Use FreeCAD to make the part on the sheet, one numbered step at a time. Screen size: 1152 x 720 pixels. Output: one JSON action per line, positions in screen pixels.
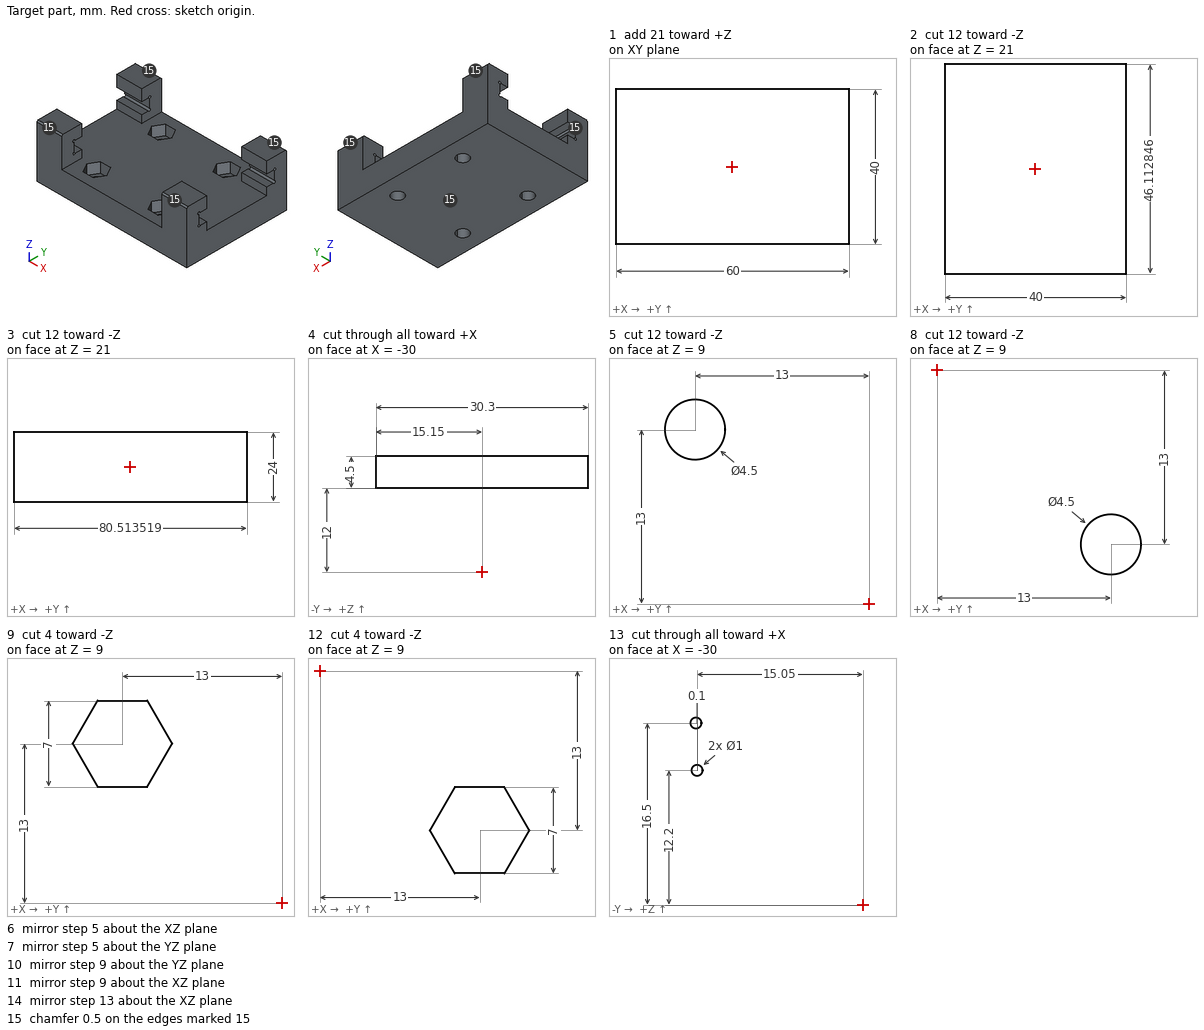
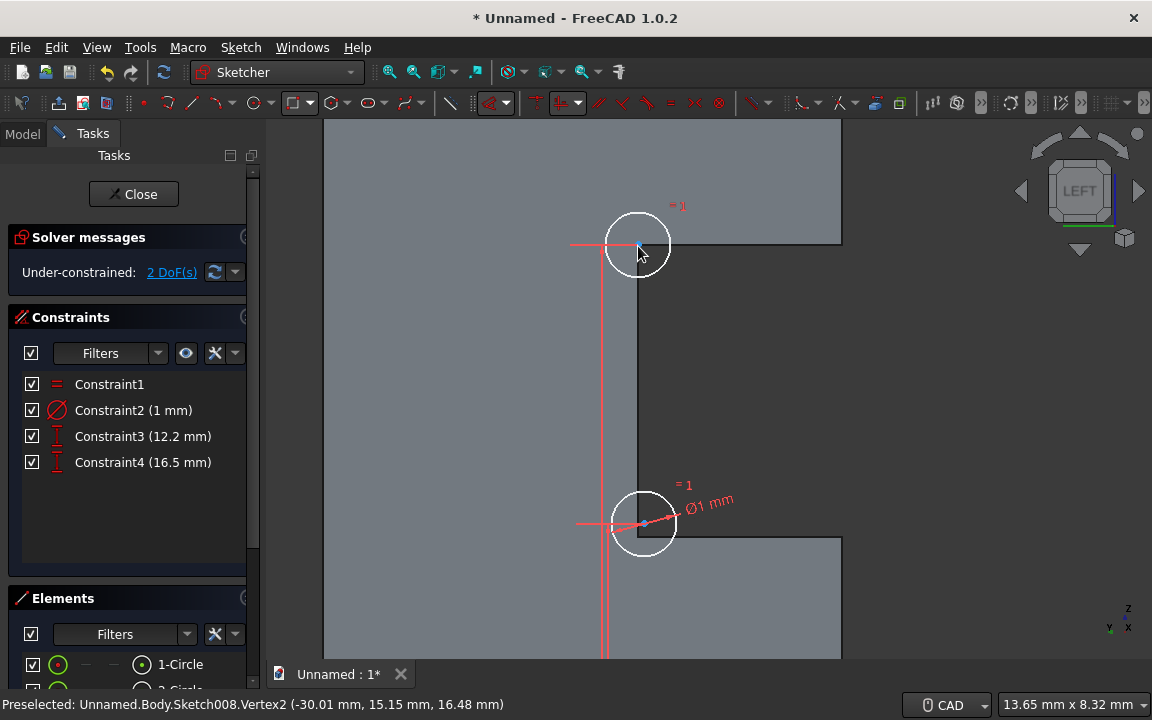
{"action": "scroll", "coordinate": [644, 524], "scroll_direction": "up", "scroll_amount": 10}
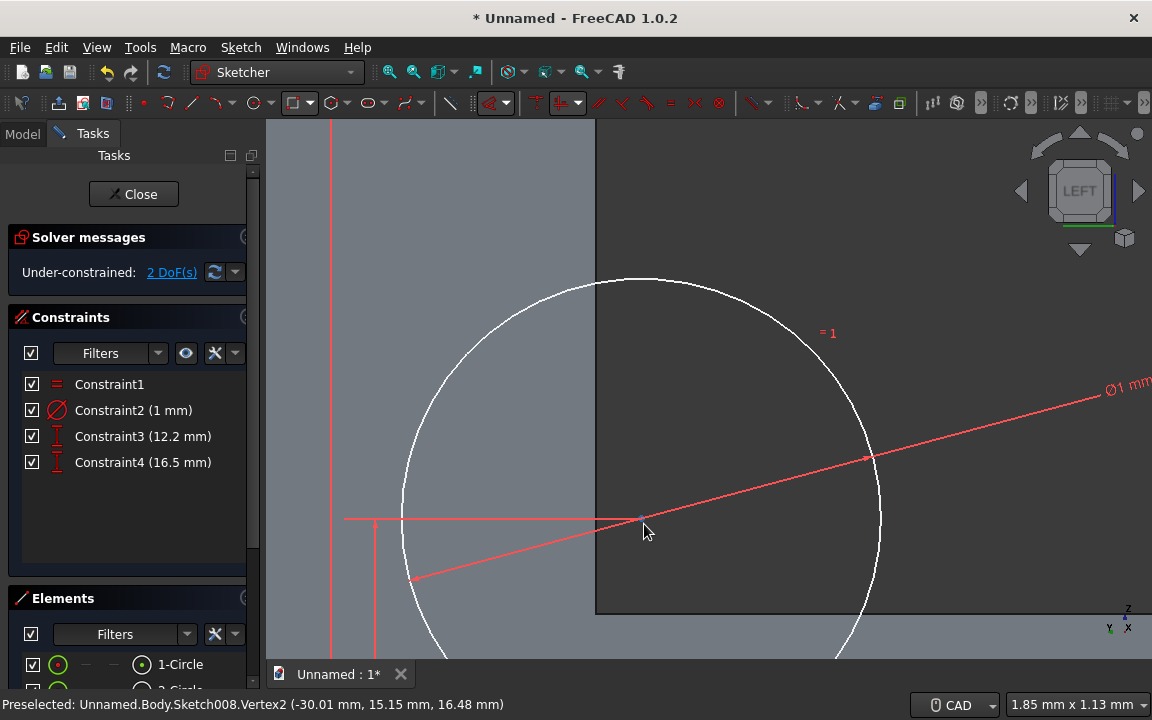
{"action": "left_click", "coordinate": [641, 519]}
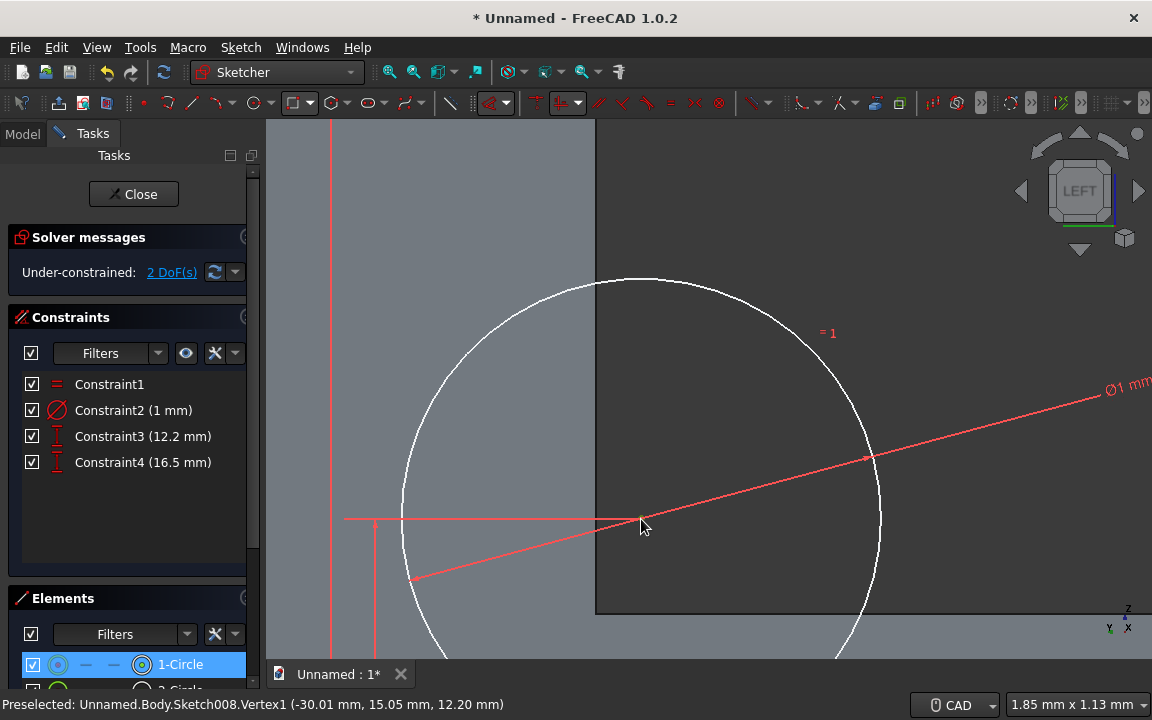
{"action": "scroll", "coordinate": [644, 530], "scroll_direction": "down", "scroll_amount": 10}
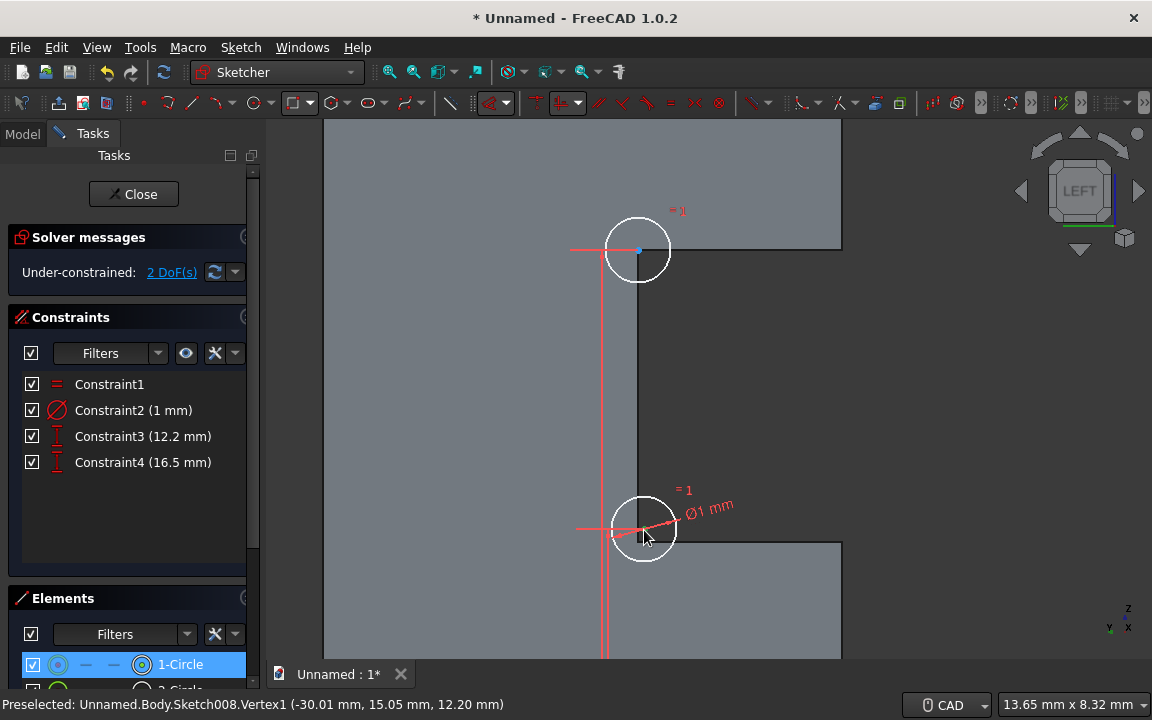
{"action": "scroll", "coordinate": [638, 250], "scroll_direction": "up", "scroll_amount": 10}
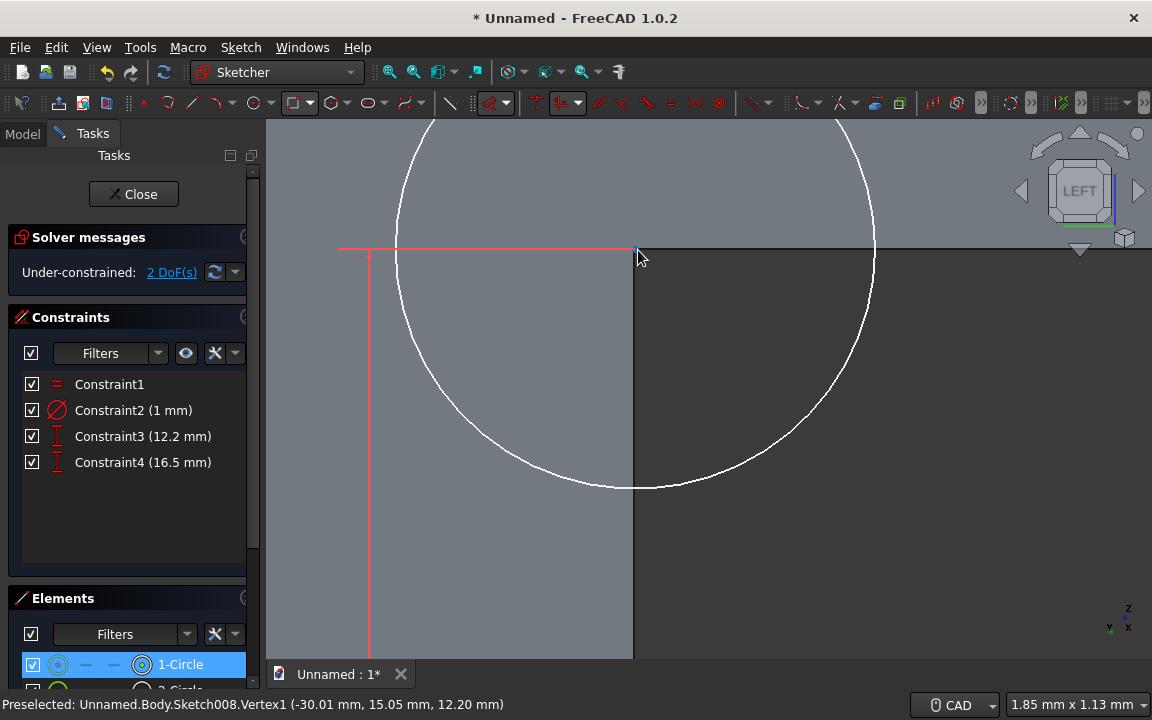
{"action": "left_click", "coordinate": [635, 249]}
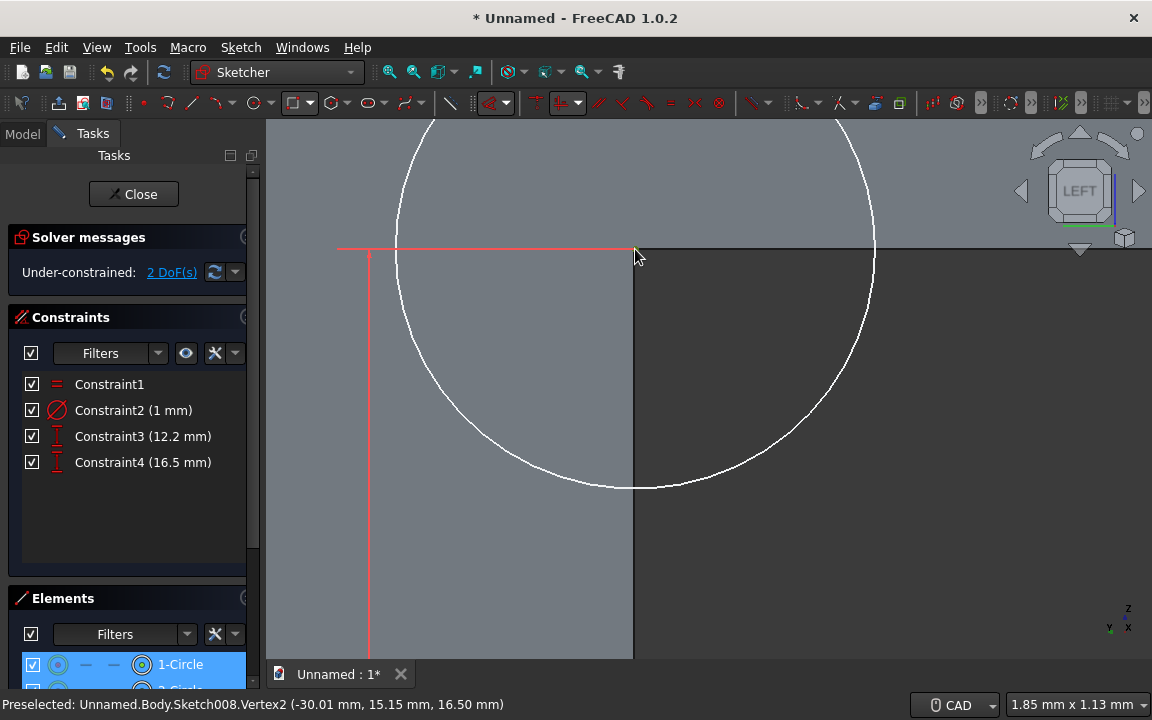
{"action": "key", "text": "l"}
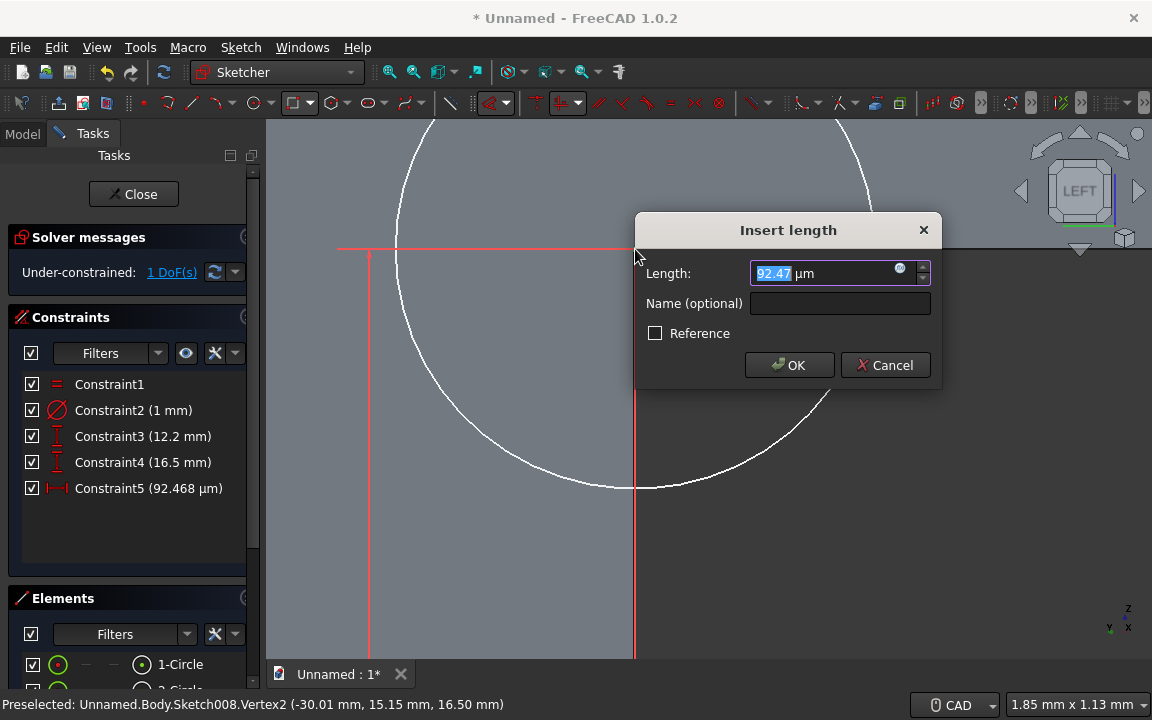
{"action": "key", "text": "ctrl+a"}
{"action": "type", "text": "0.1 mm"}
{"action": "key", "text": "Return"}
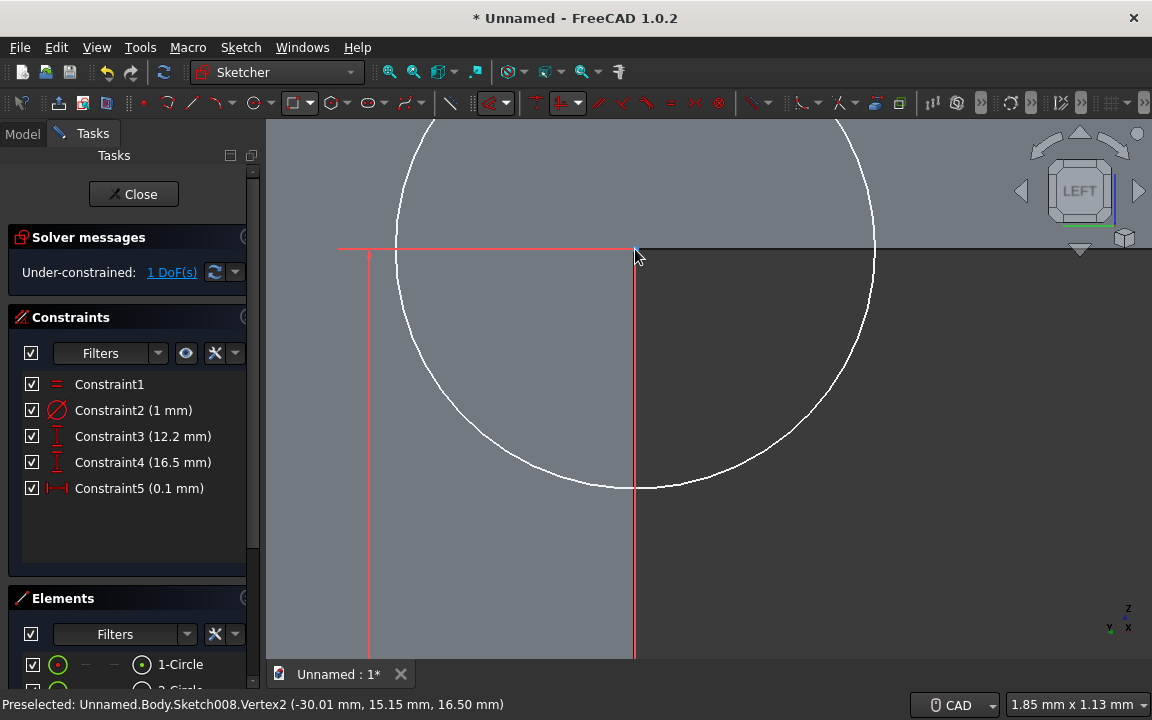
{"action": "scroll", "coordinate": [638, 250], "scroll_direction": "down", "scroll_amount": 10}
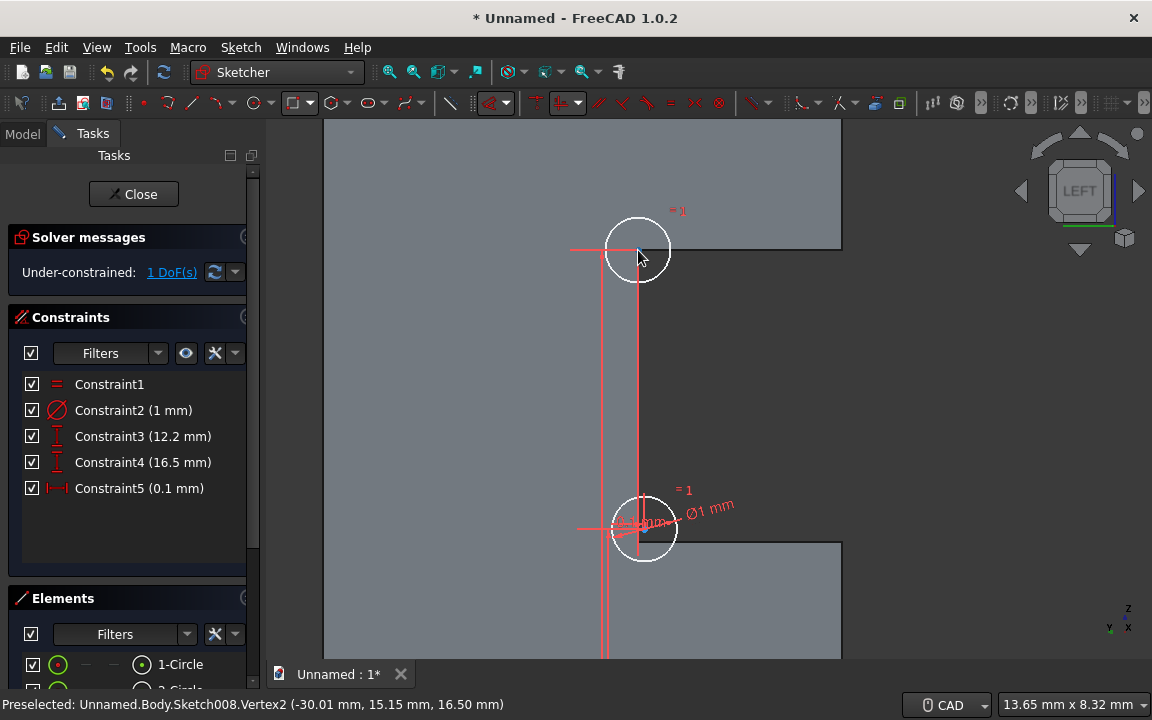
{"action": "left_click", "coordinate": [644, 529]}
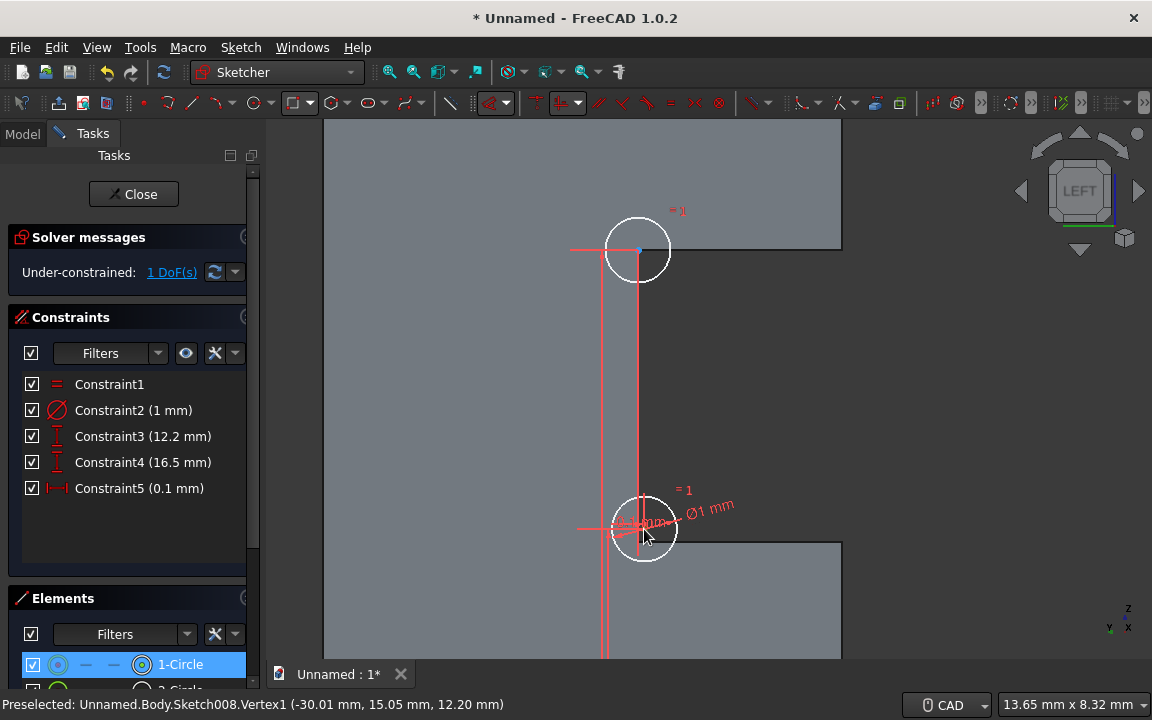
{"action": "left_click", "coordinate": [508, 104]}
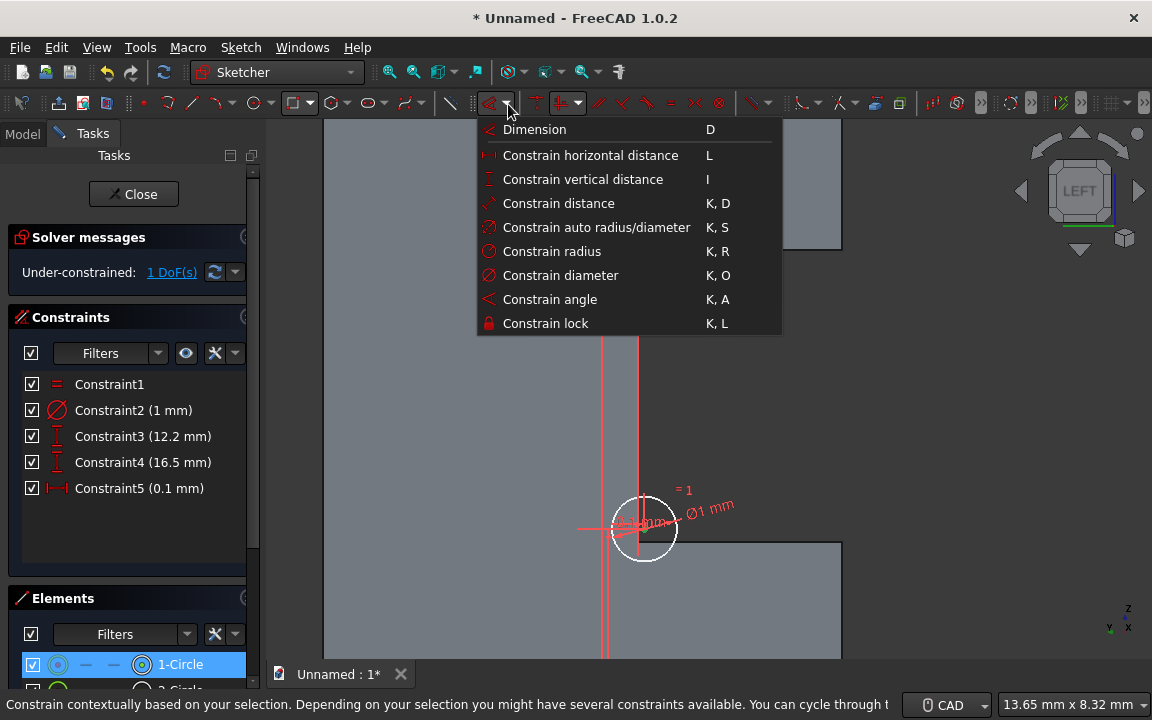
{"action": "left_click", "coordinate": [630, 155]}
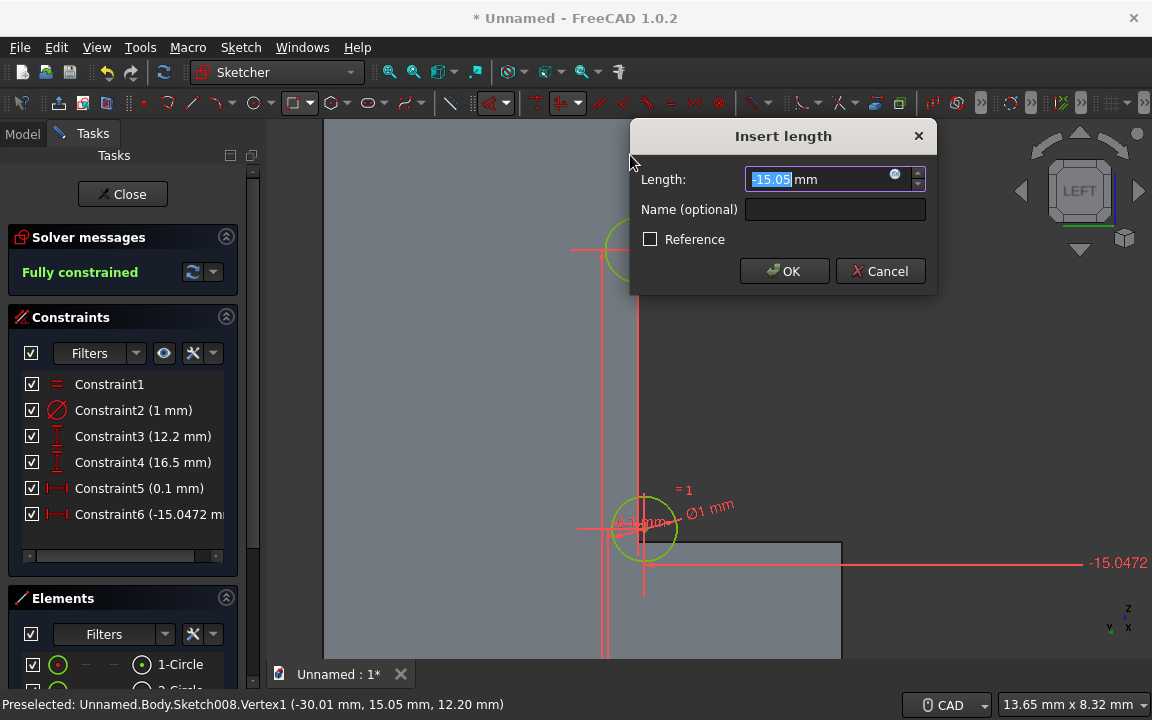
{"action": "type", "text": "-15.05"}
{"action": "key", "text": "Return"}